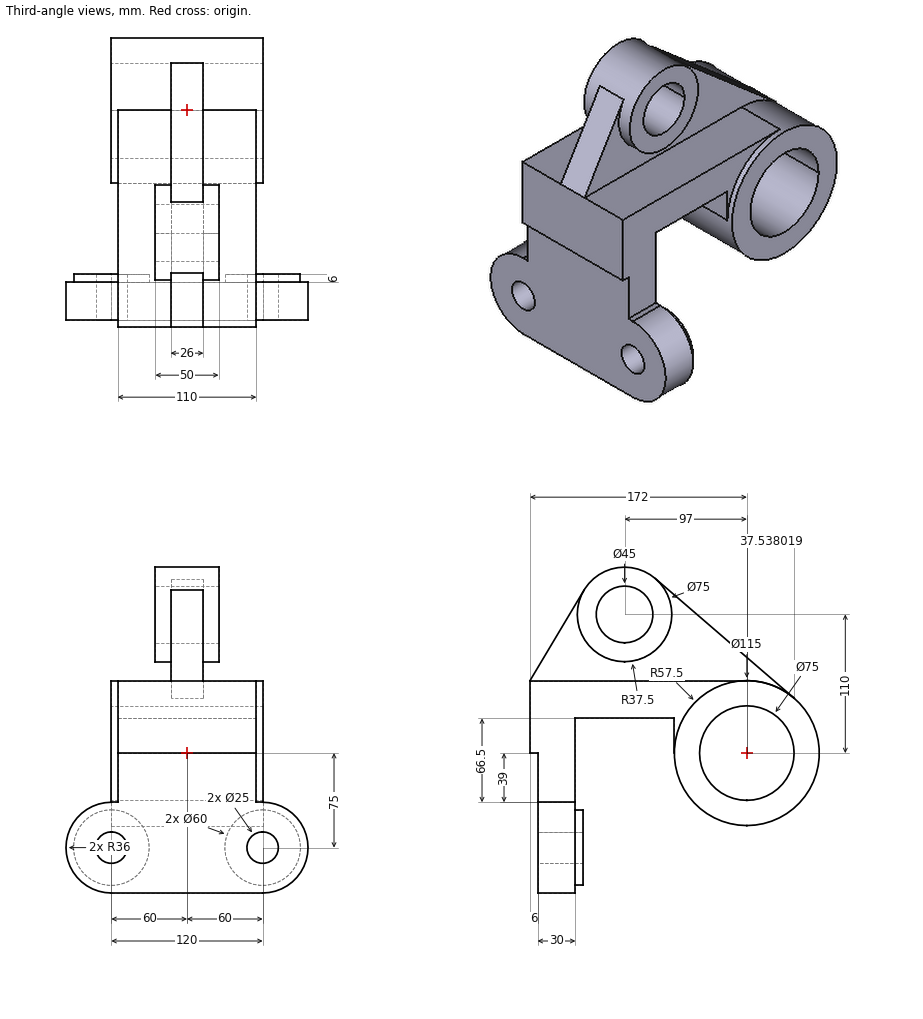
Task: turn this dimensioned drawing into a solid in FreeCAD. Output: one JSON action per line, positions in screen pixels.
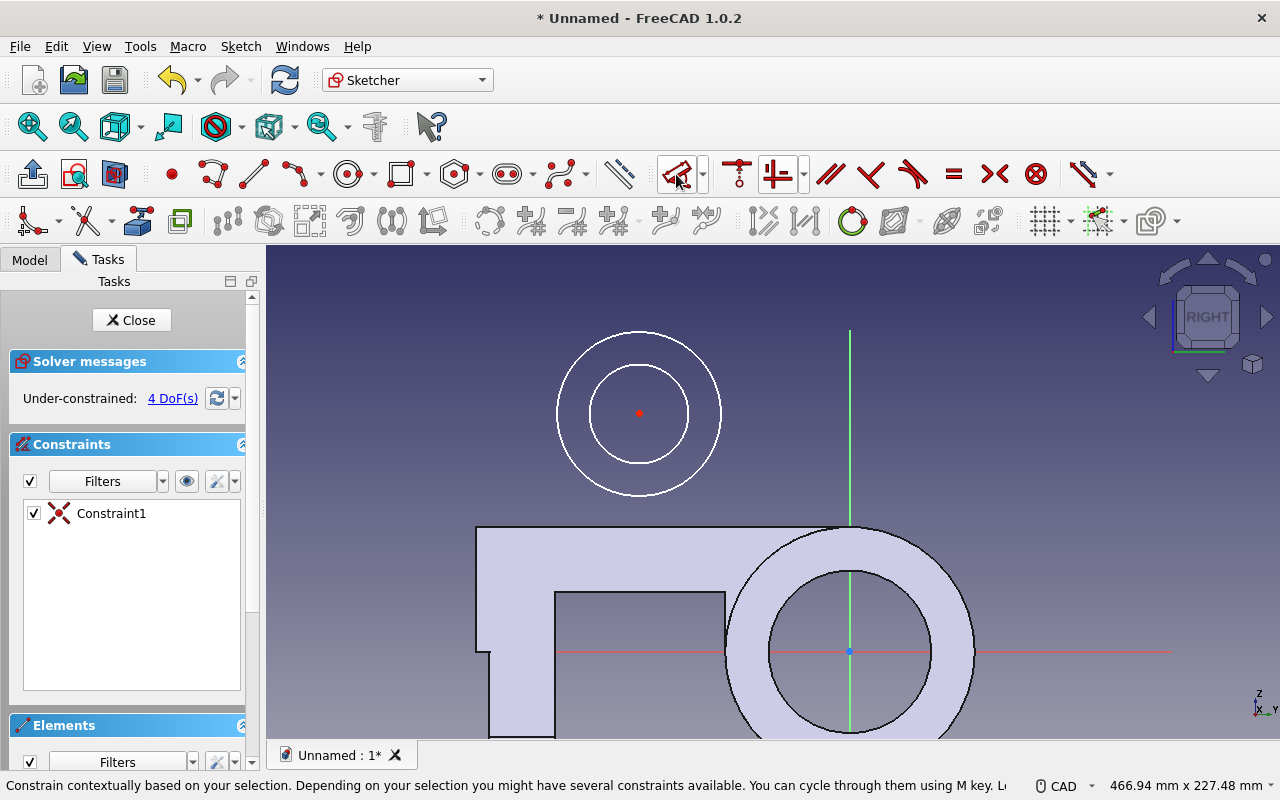
{"action": "left_click", "coordinate": [697, 356]}
{"action": "left_click", "coordinate": [720, 333]}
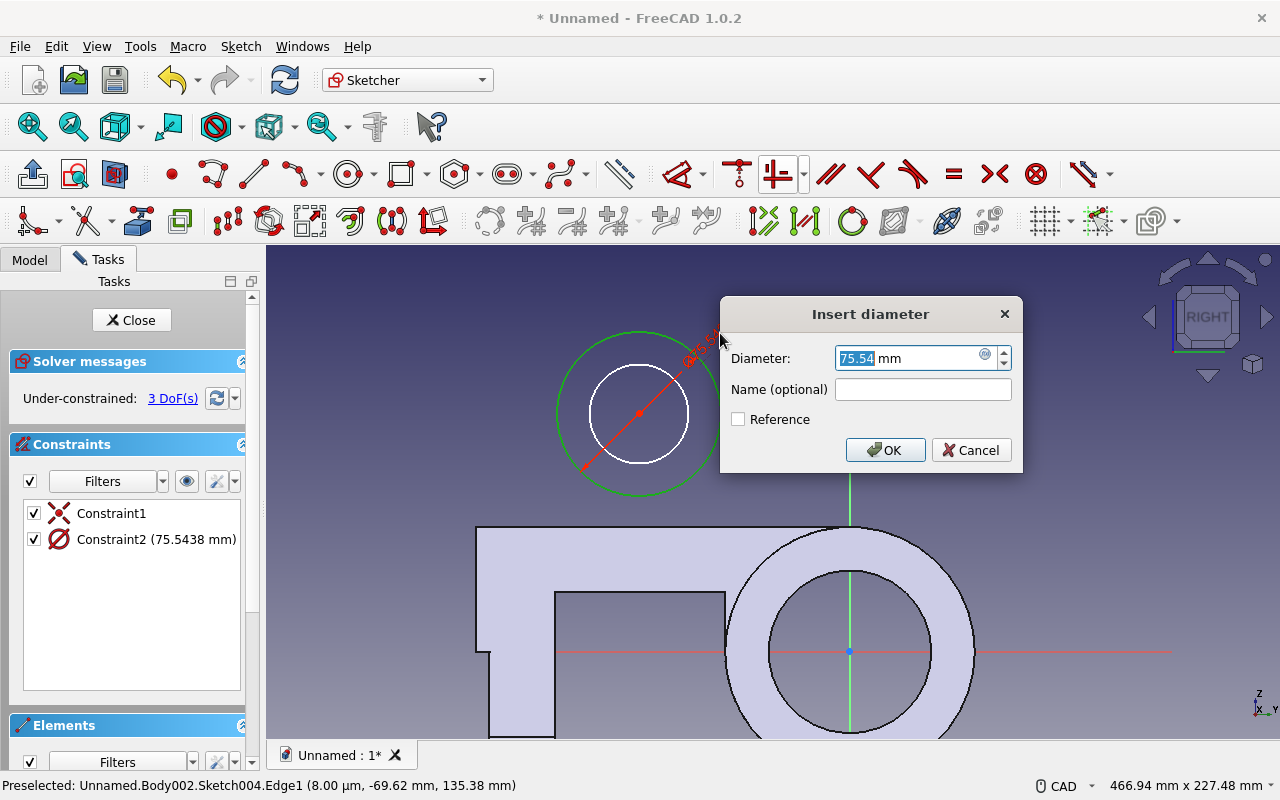
{"action": "type", "text": "75"}
{"action": "key", "text": "Return"}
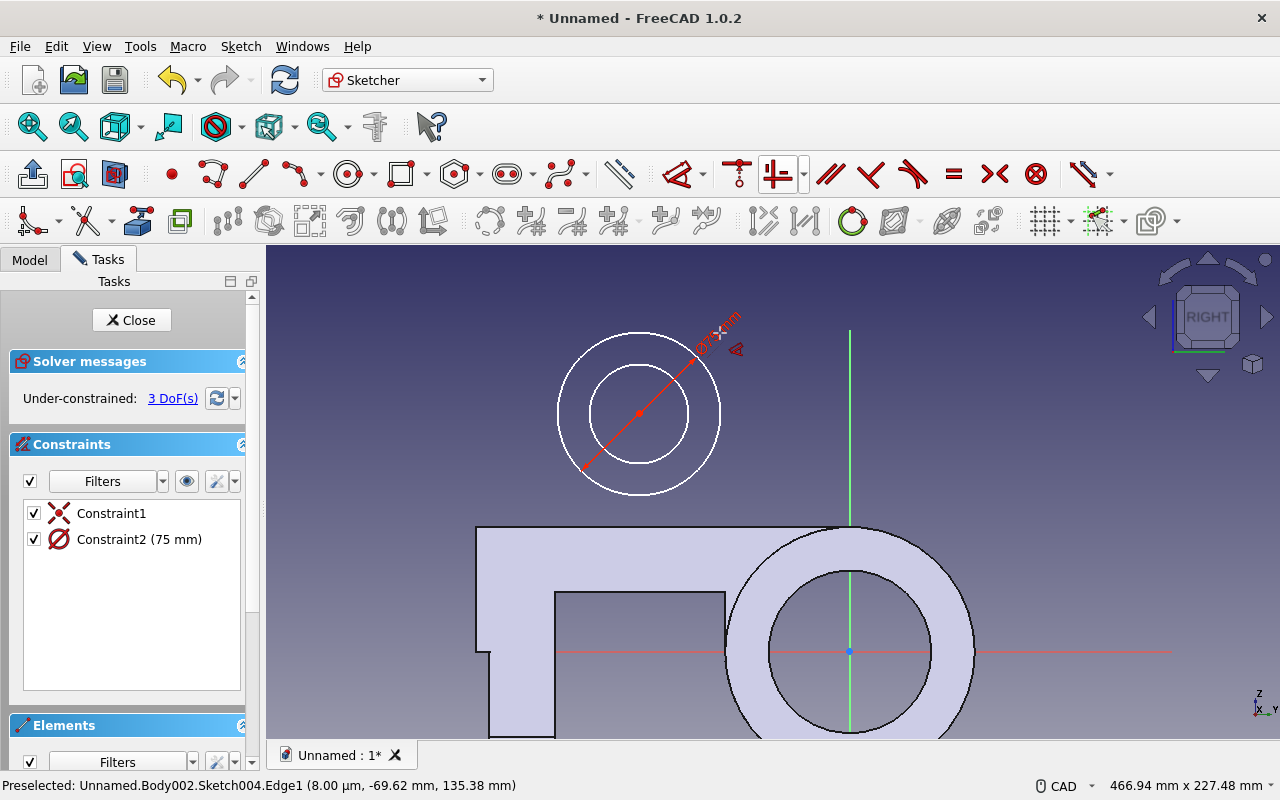
{"action": "left_click", "coordinate": [674, 379]}
{"action": "left_click", "coordinate": [739, 385]}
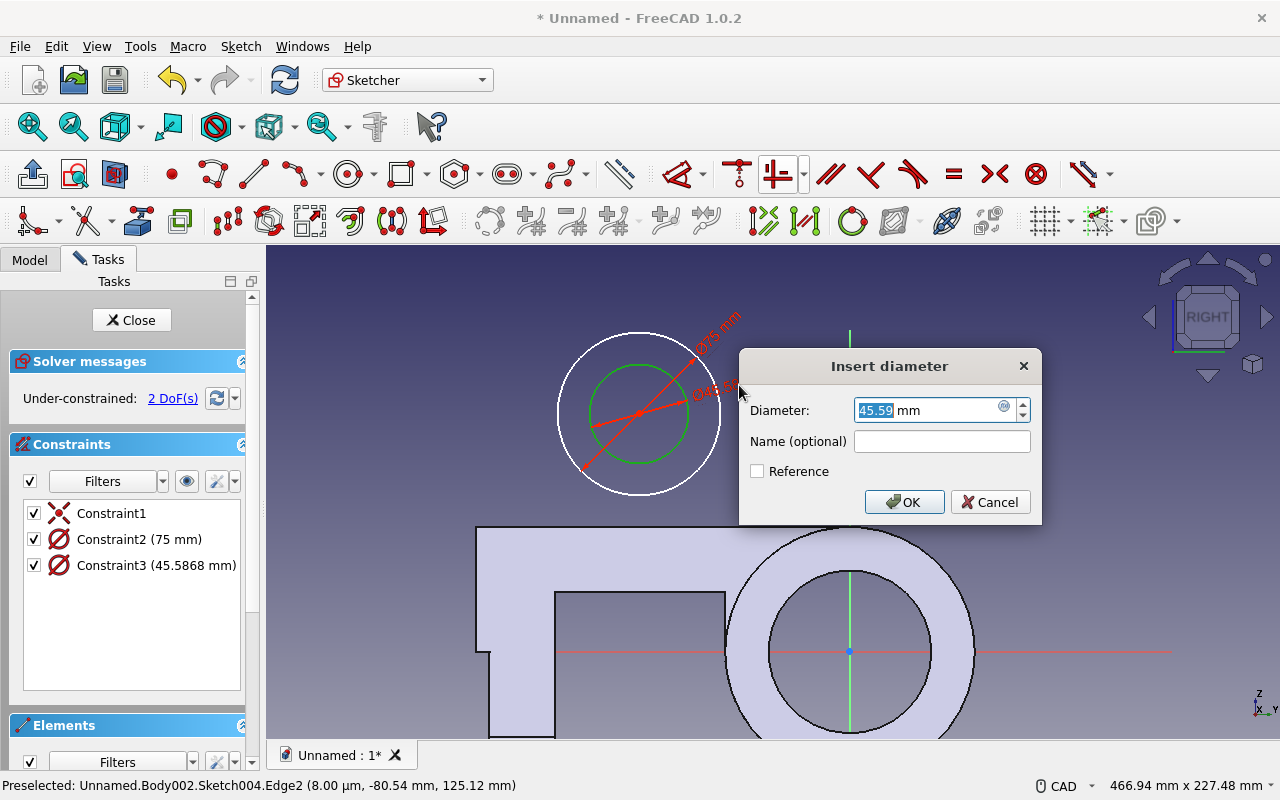
{"action": "type", "text": "45"}
{"action": "key", "text": "Return"}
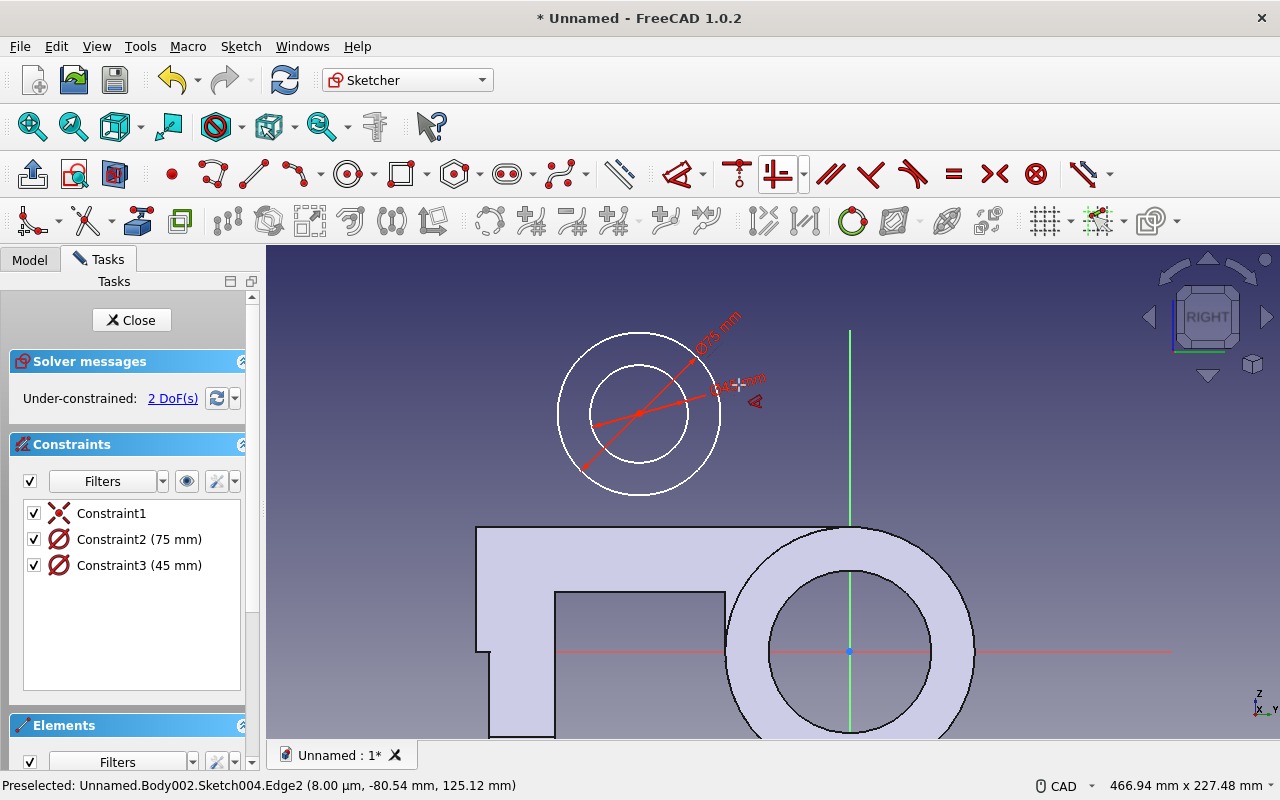
{"action": "left_click", "coordinate": [639, 414]}
{"action": "left_click", "coordinate": [744, 686]}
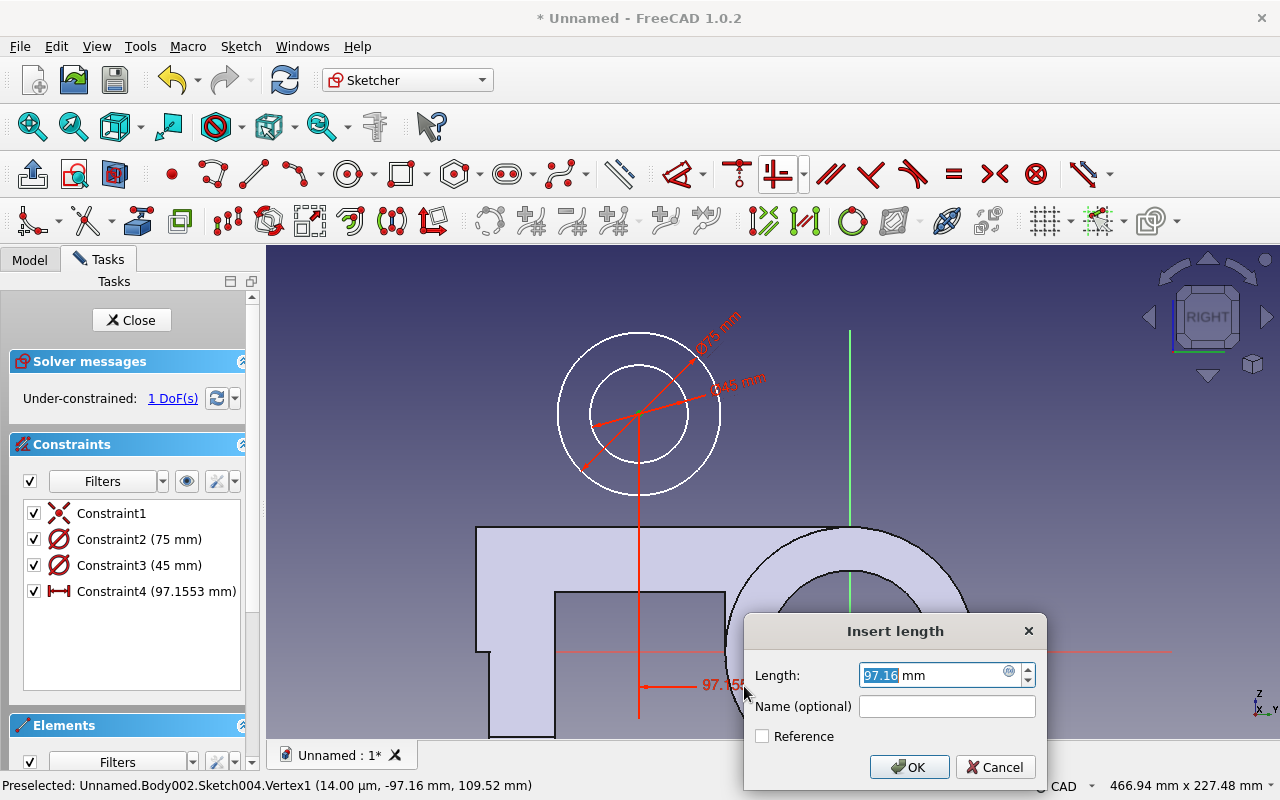
{"action": "type", "text": "97"}
{"action": "key", "text": "Return"}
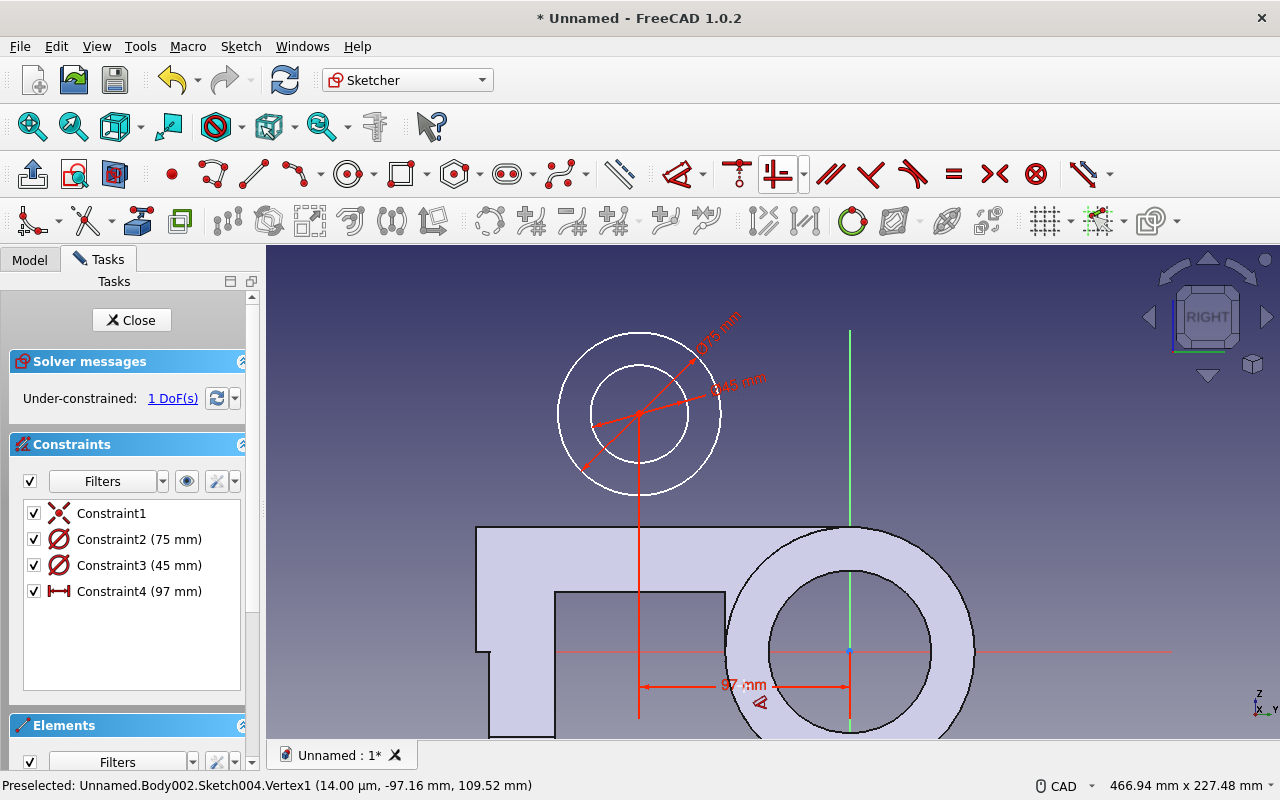
{"action": "left_click", "coordinate": [639, 414]}
{"action": "left_click", "coordinate": [884, 533]}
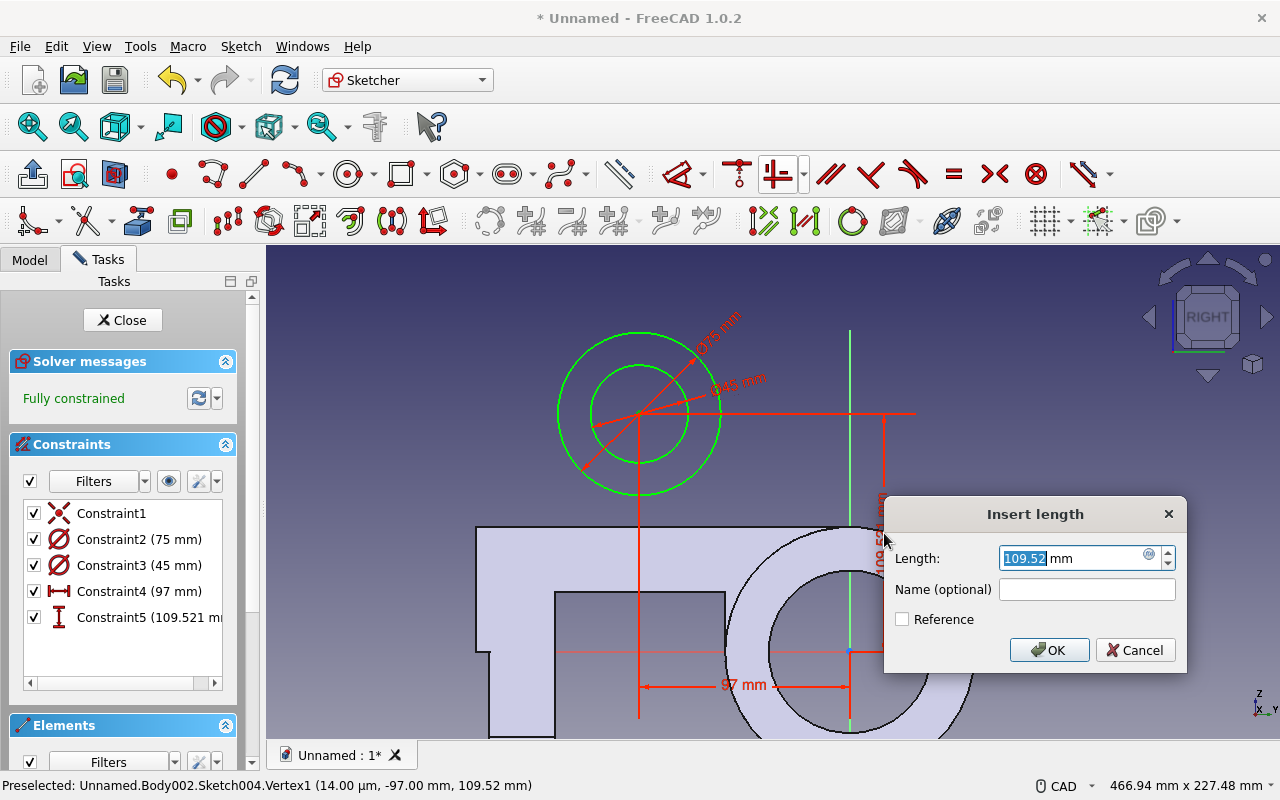
{"action": "type", "text": "110"}
{"action": "key", "text": "Return"}
{"action": "key", "text": "Escape"}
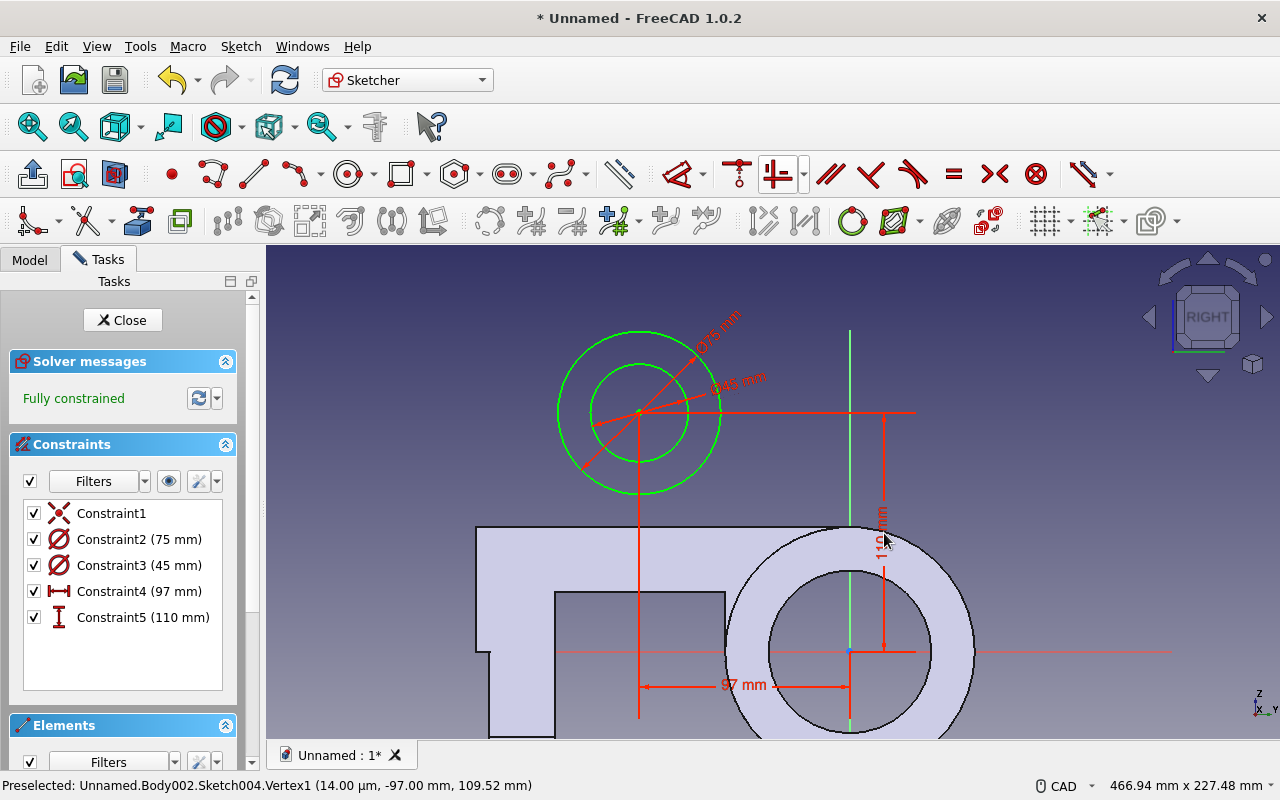
{"action": "left_click", "coordinate": [123, 320]}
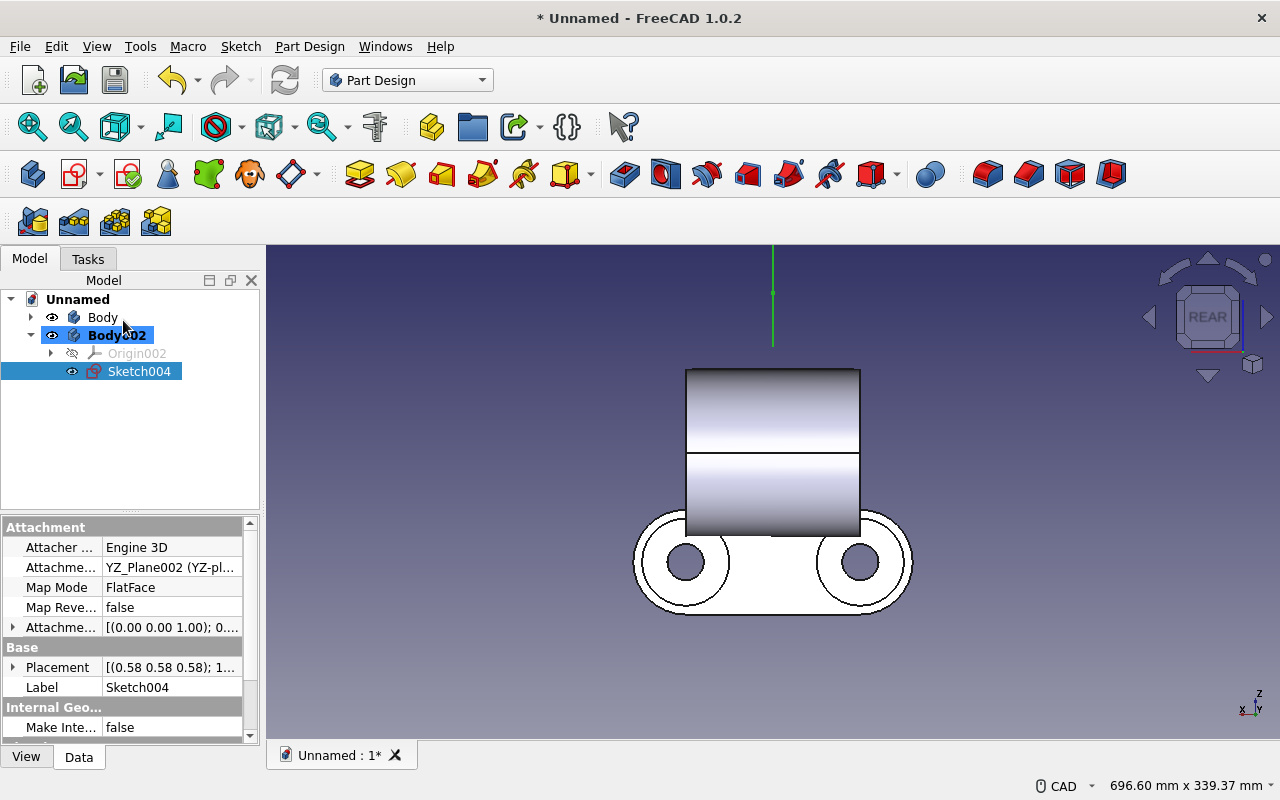
{"action": "left_click", "coordinate": [360, 174]}